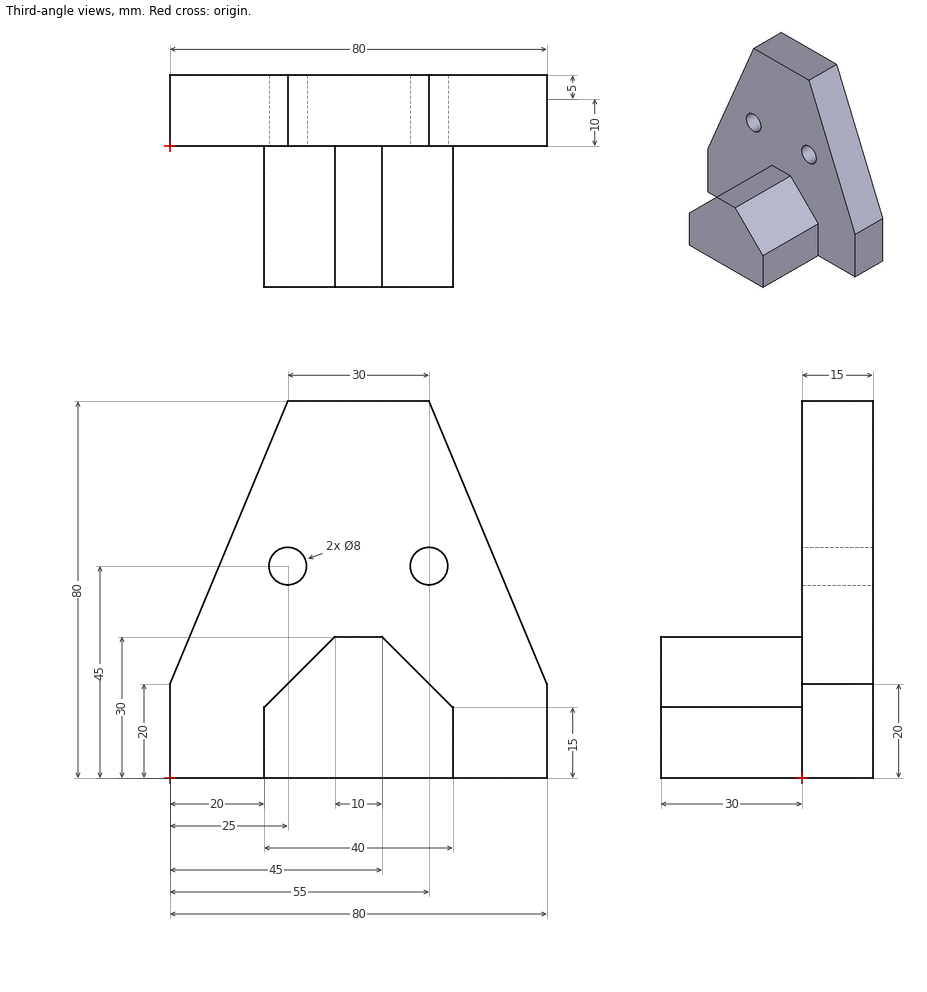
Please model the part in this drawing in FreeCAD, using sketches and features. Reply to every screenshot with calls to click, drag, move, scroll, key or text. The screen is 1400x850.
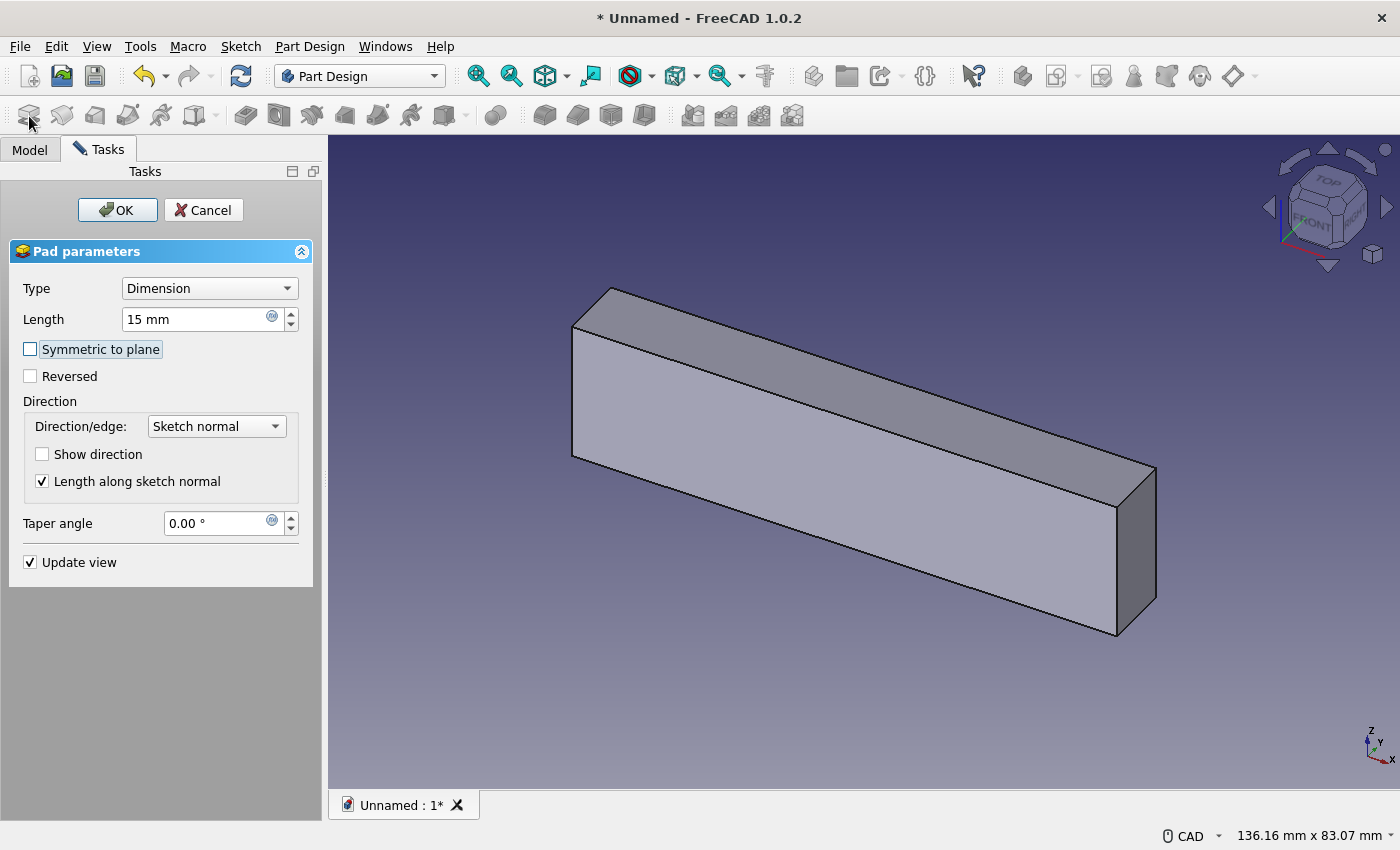
click(31, 376)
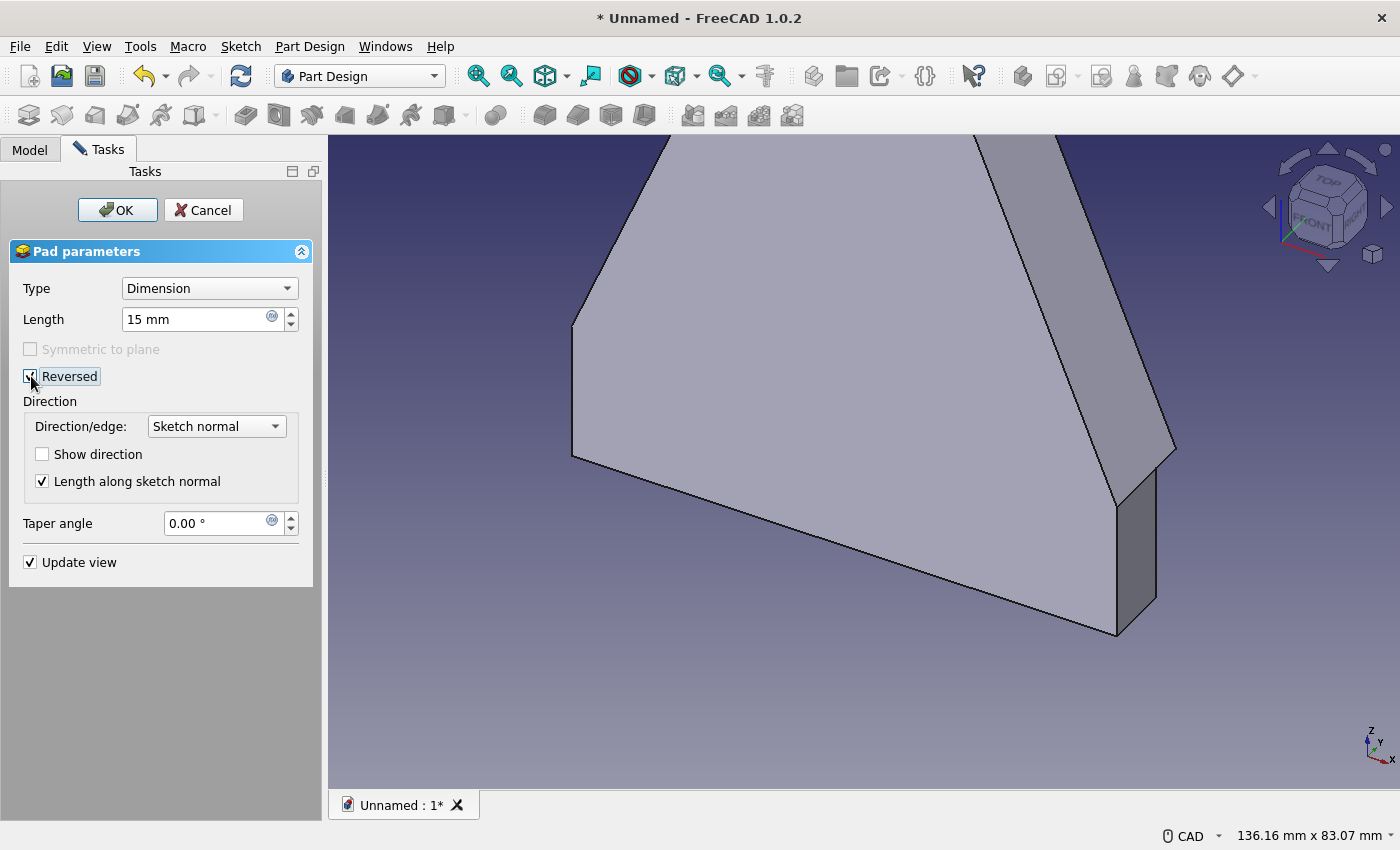
click(118, 210)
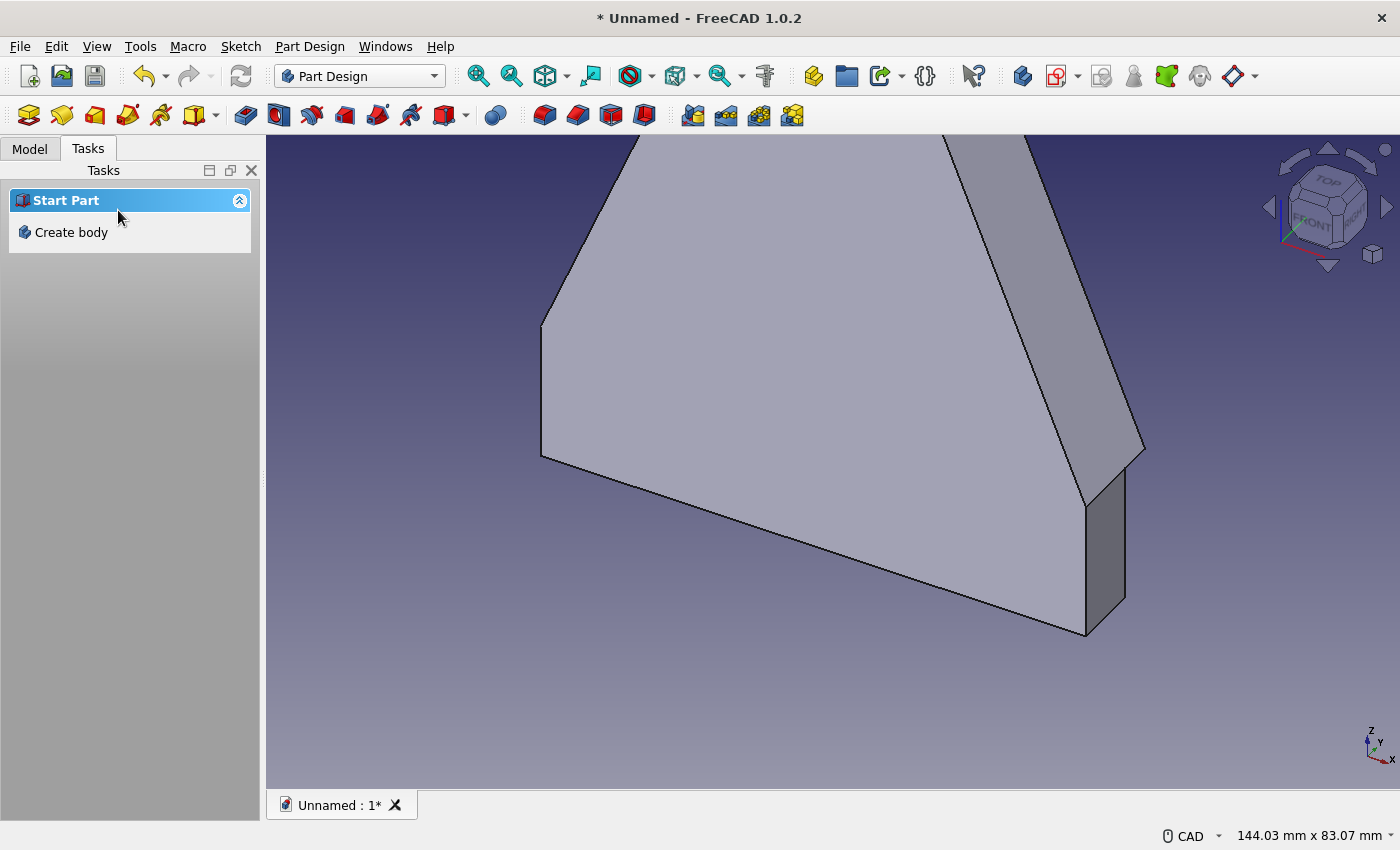
click(479, 76)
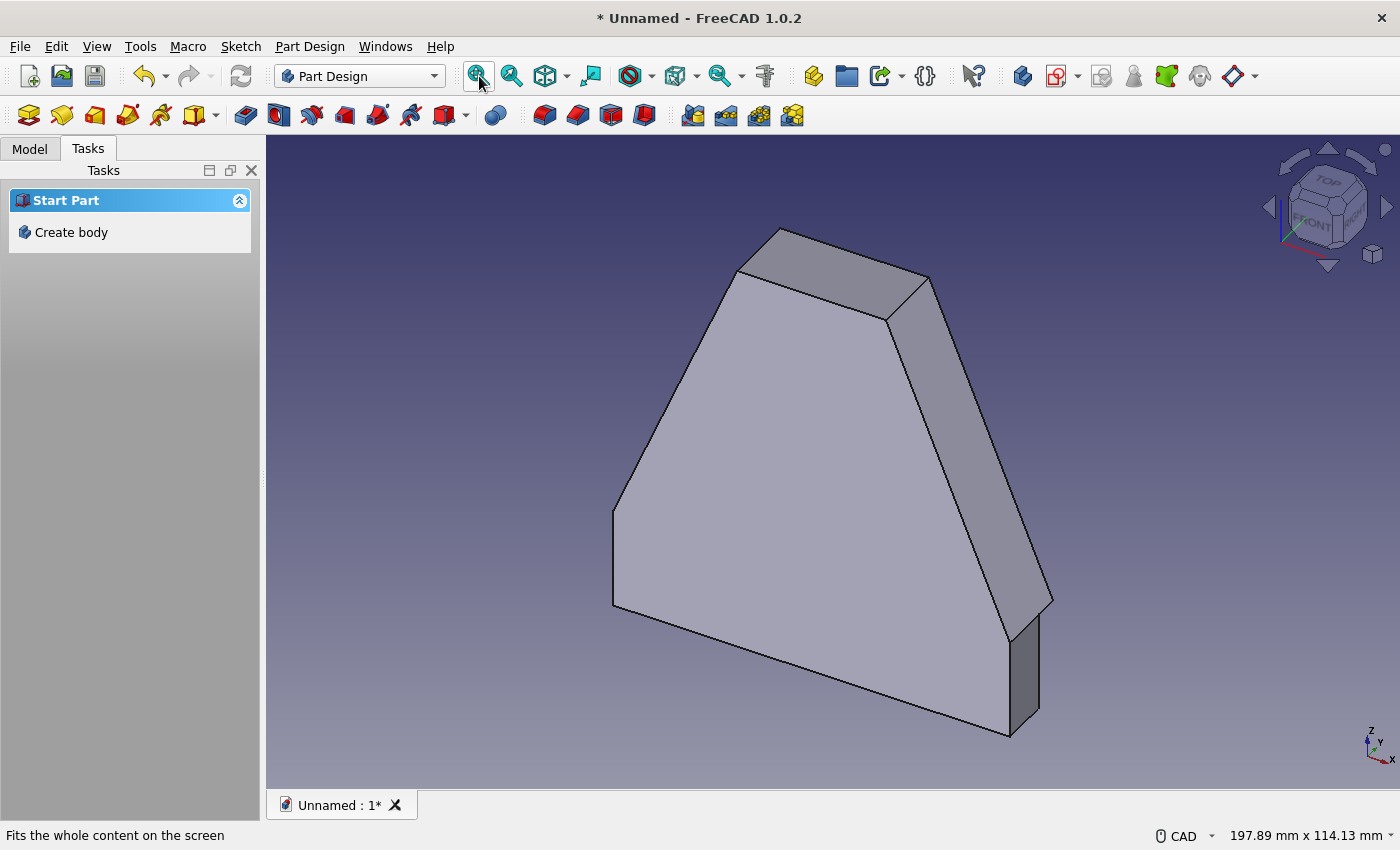
key(5)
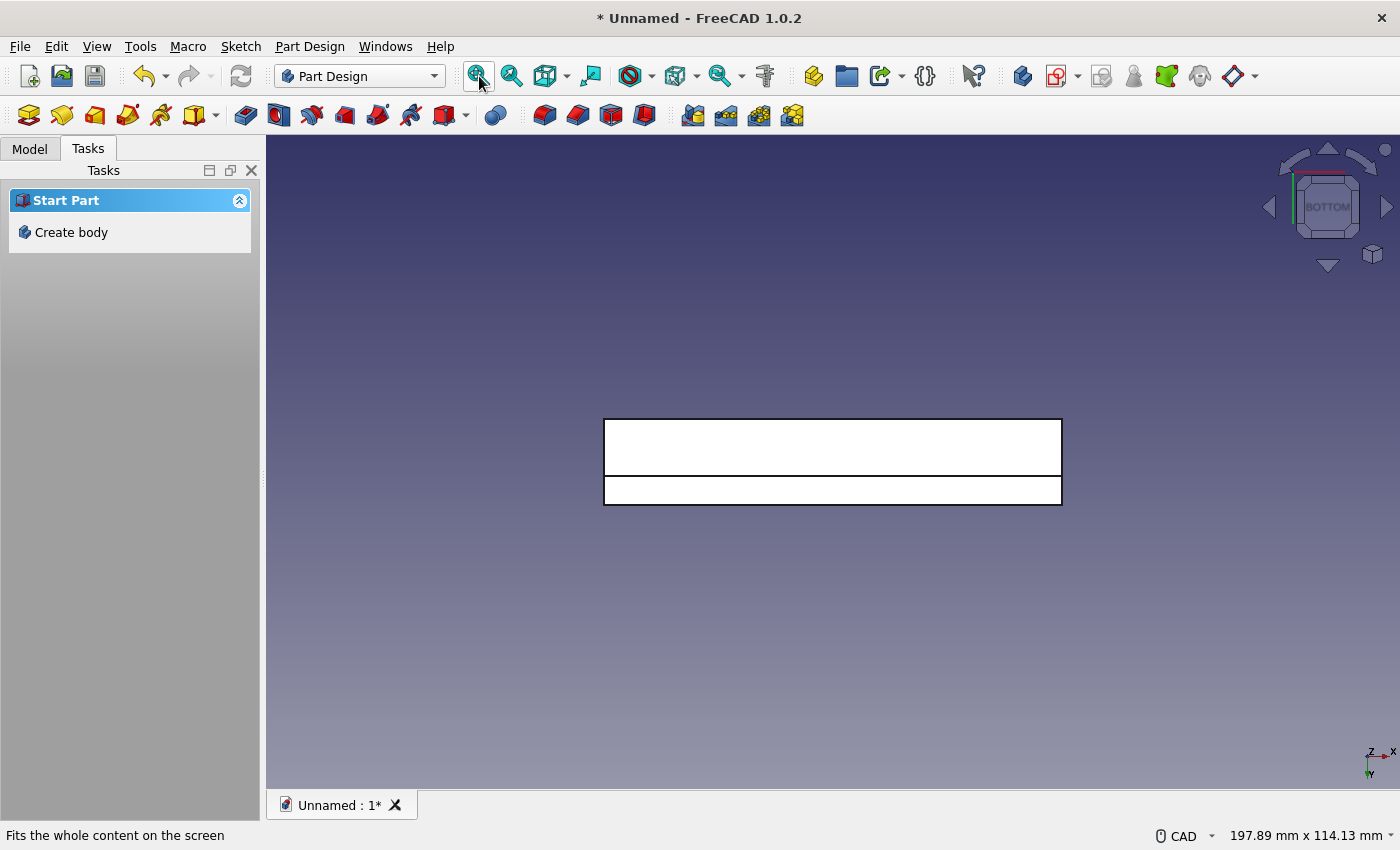
click(479, 76)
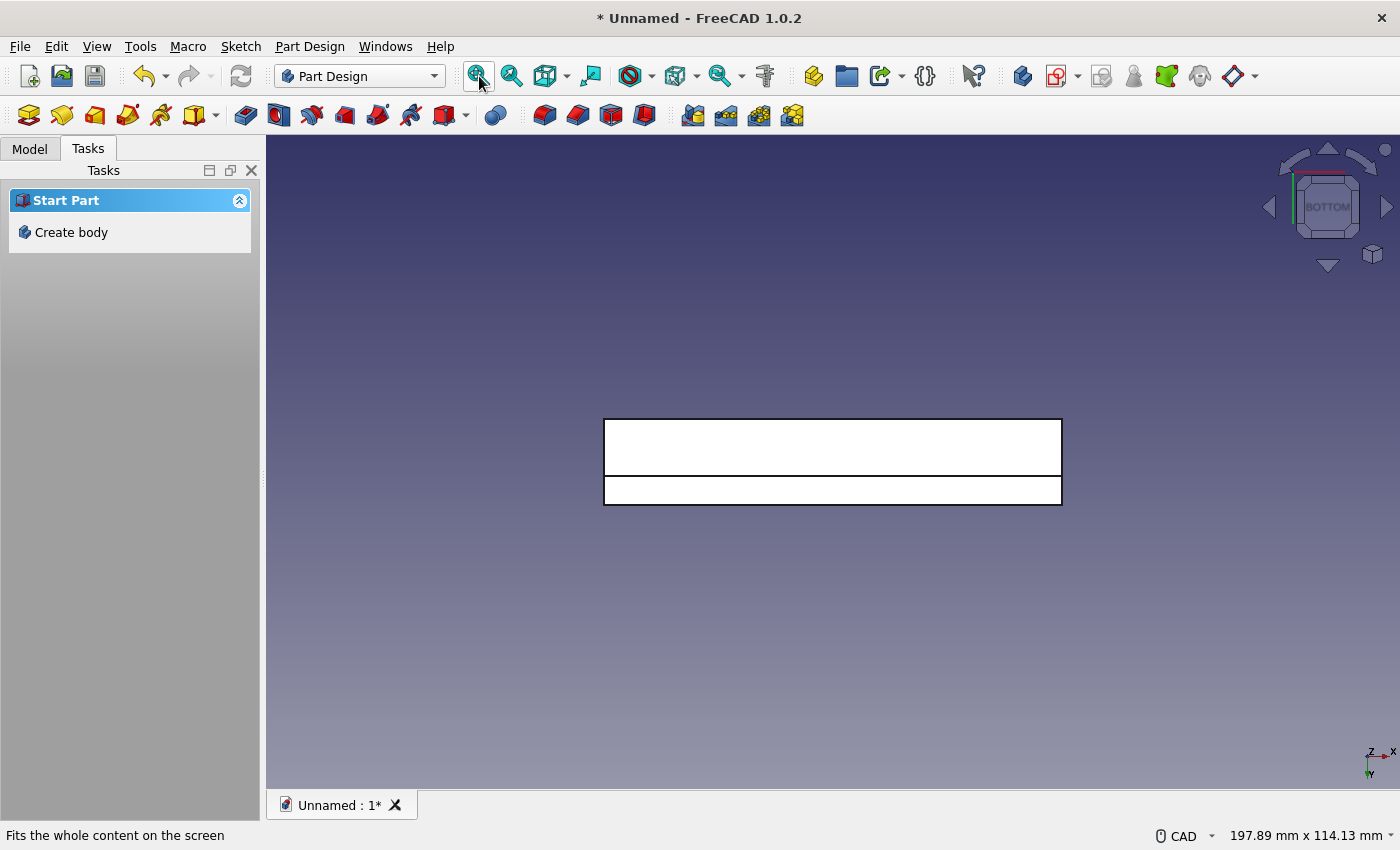
click(1029, 447)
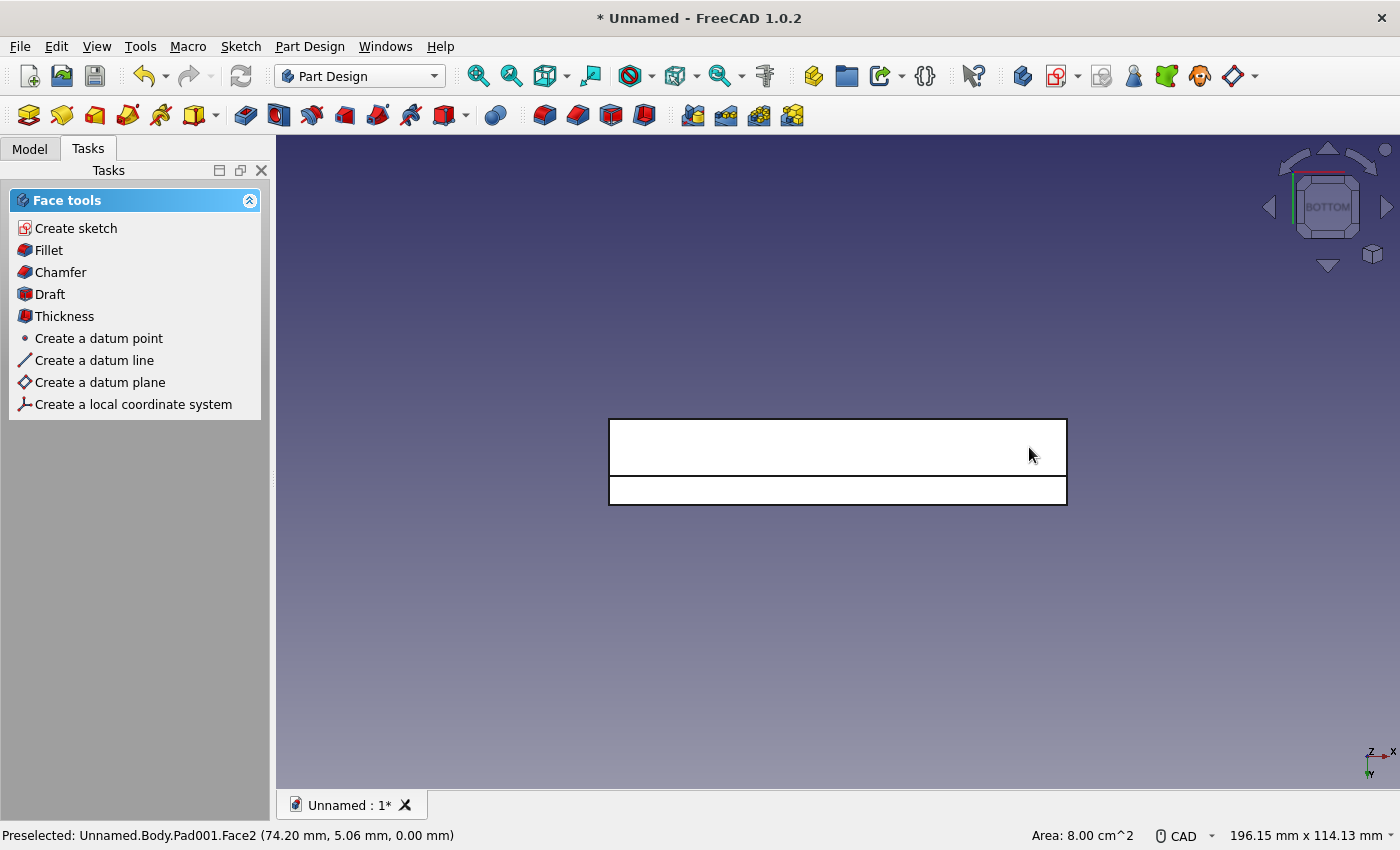
click(1056, 76)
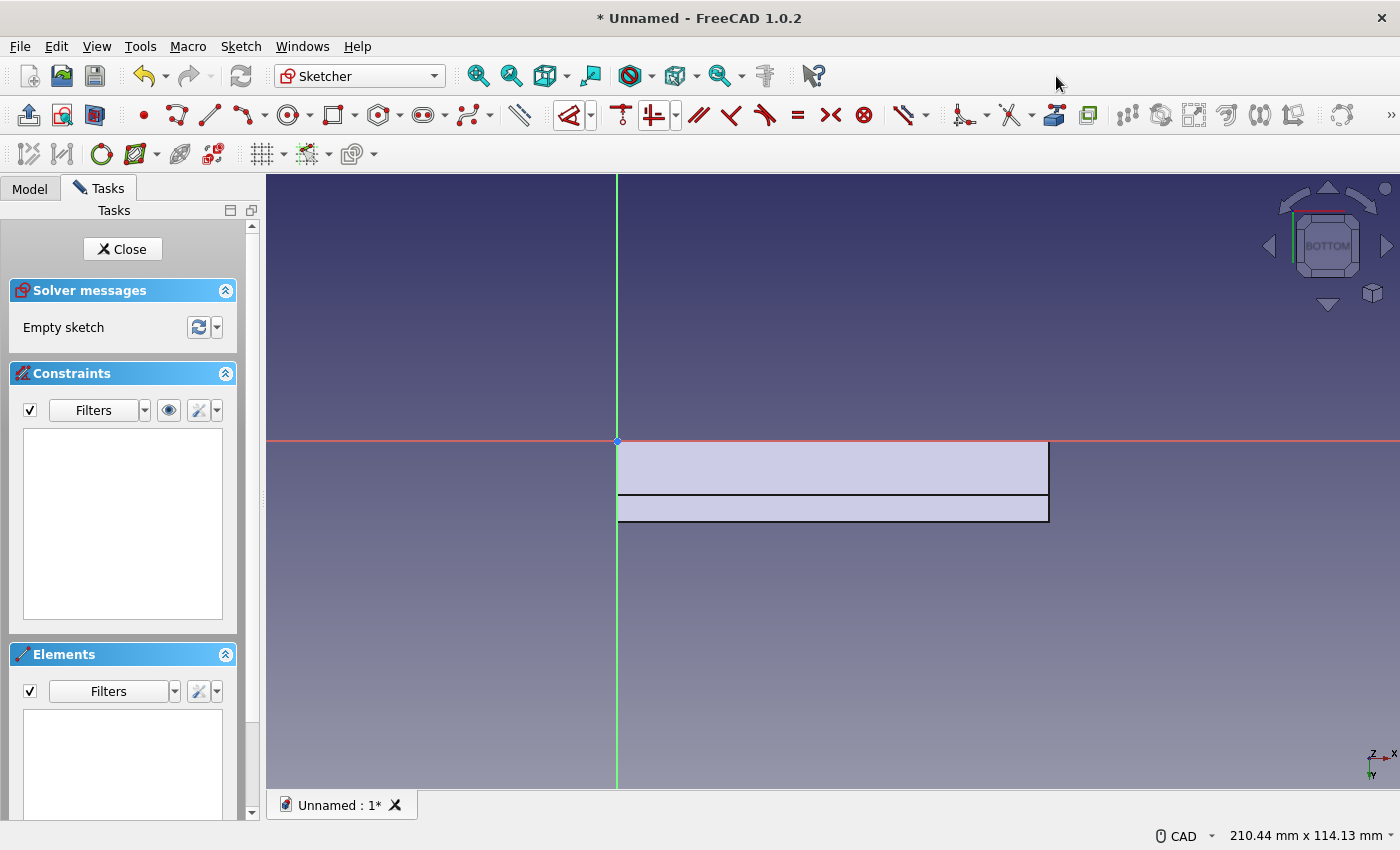
scroll(972, 482, up, 2)